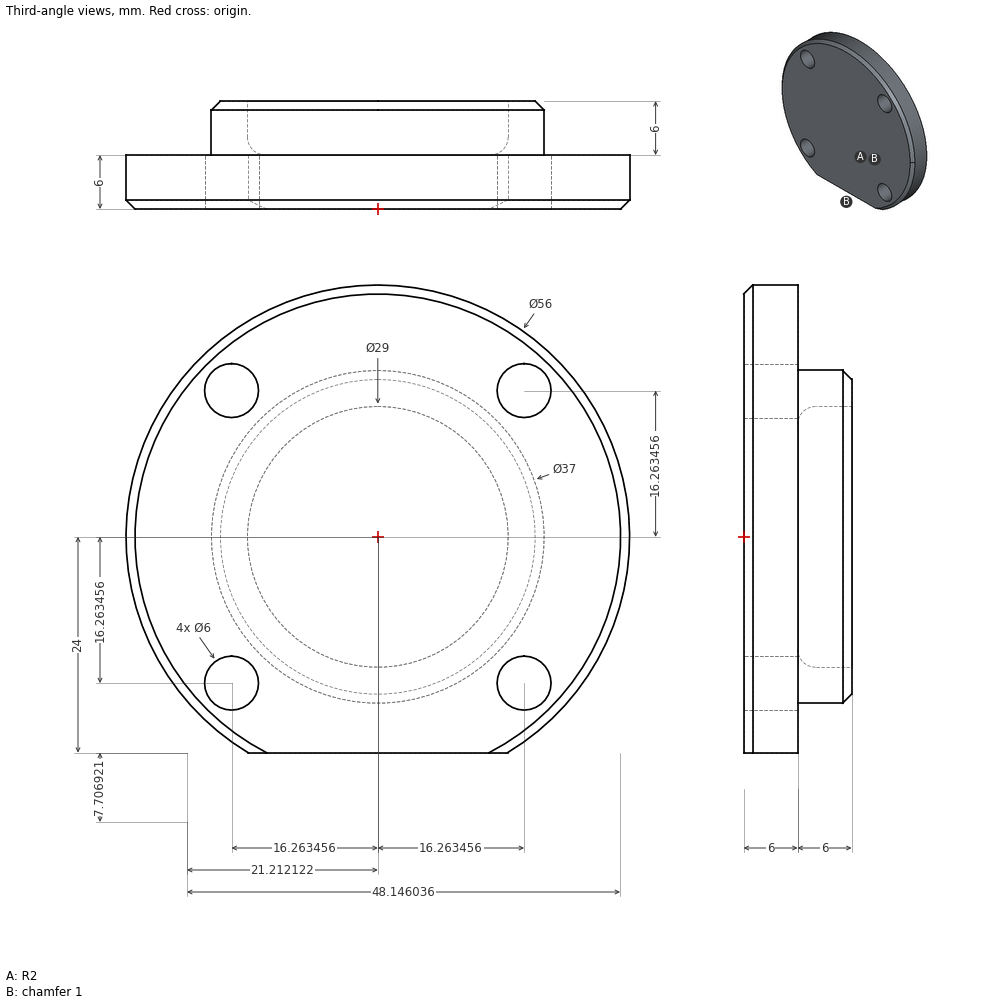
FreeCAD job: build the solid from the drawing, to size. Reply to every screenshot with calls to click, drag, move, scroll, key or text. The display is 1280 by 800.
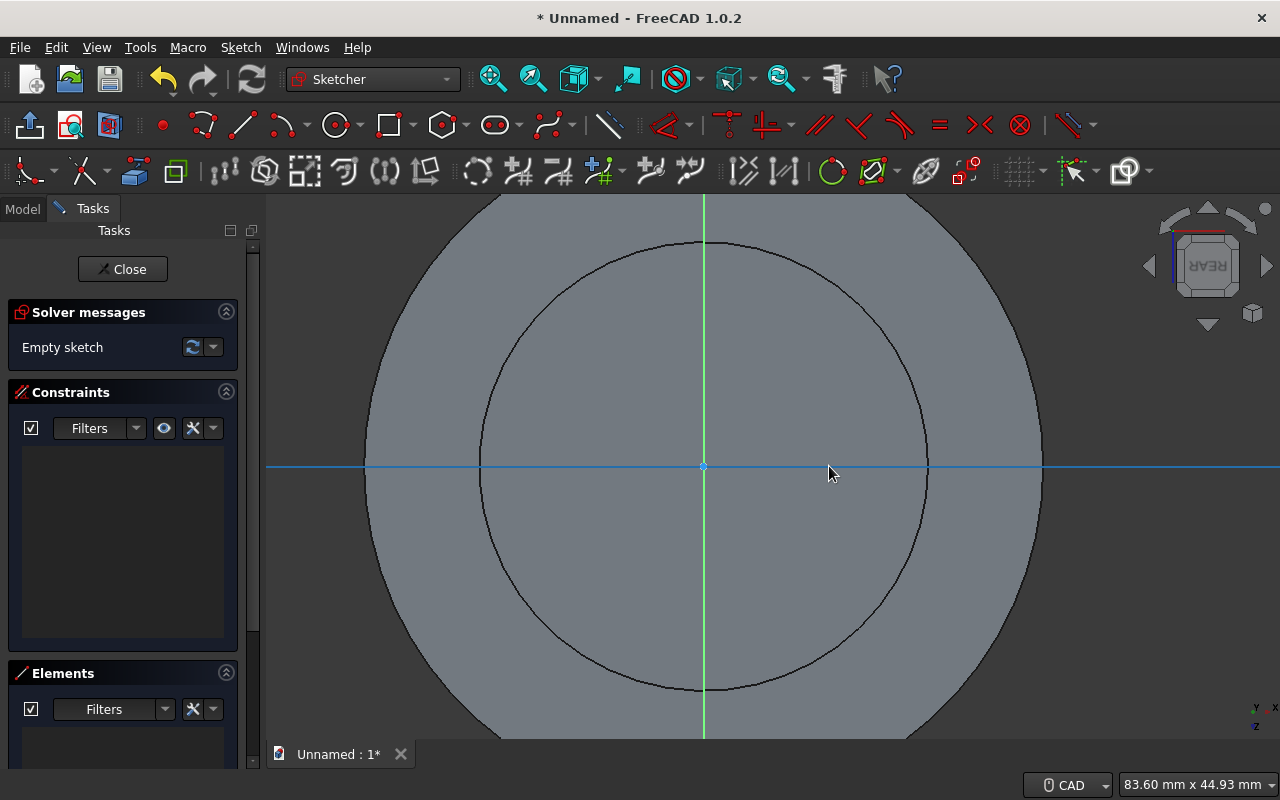
key(g)
key(c)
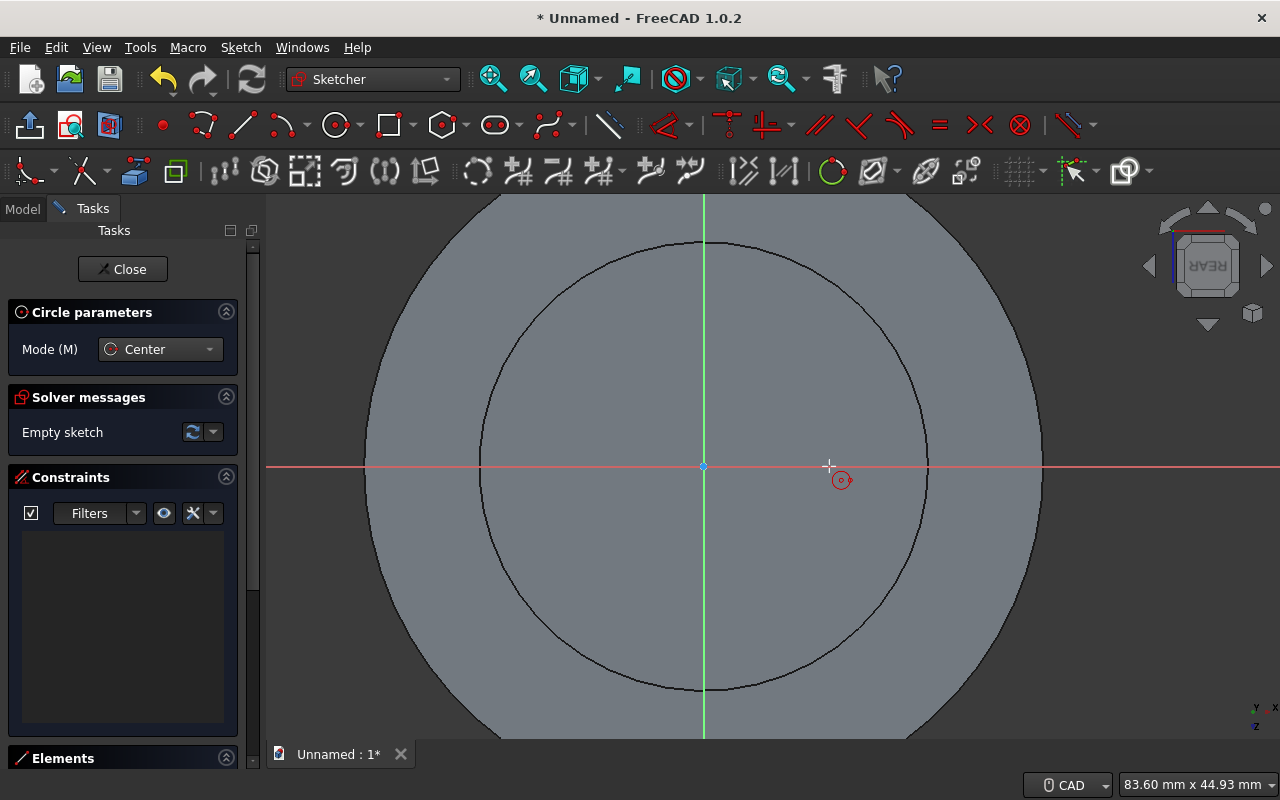
click(704, 466)
click(828, 342)
key(Escape)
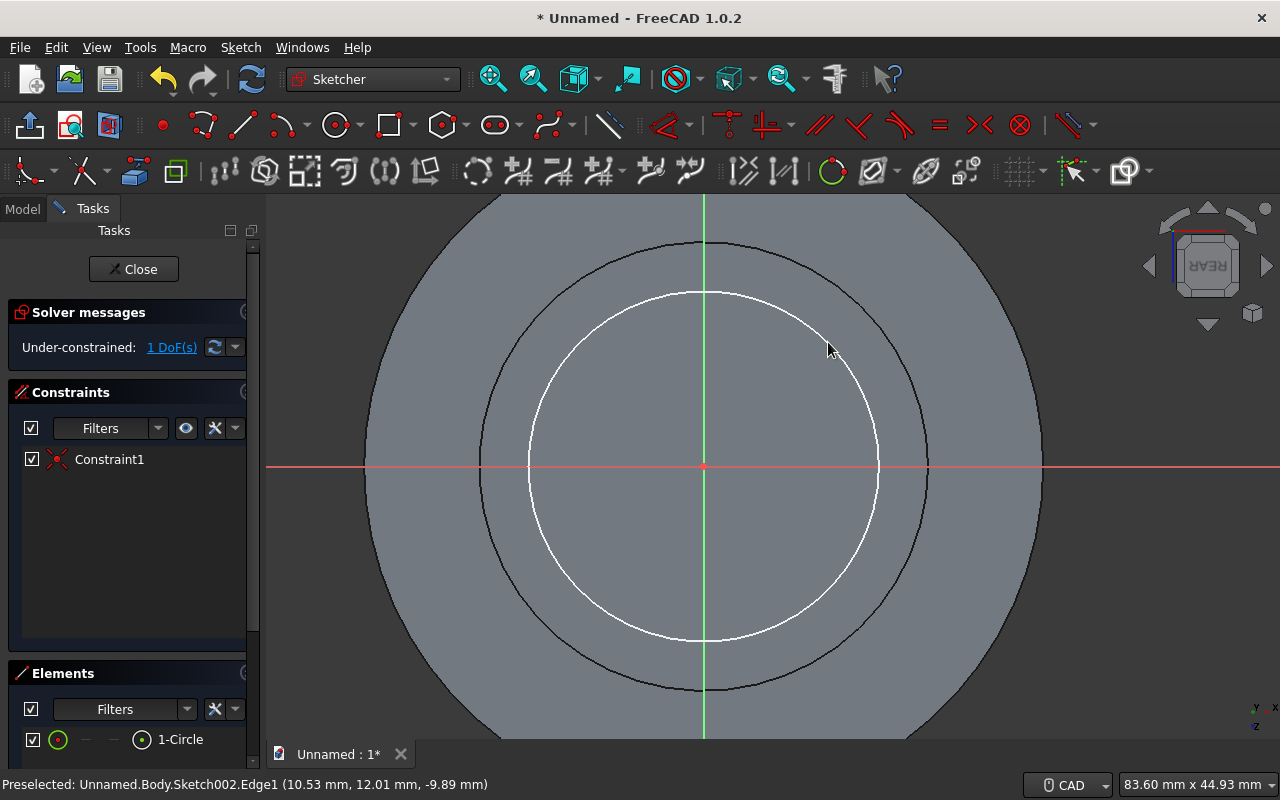
key(d)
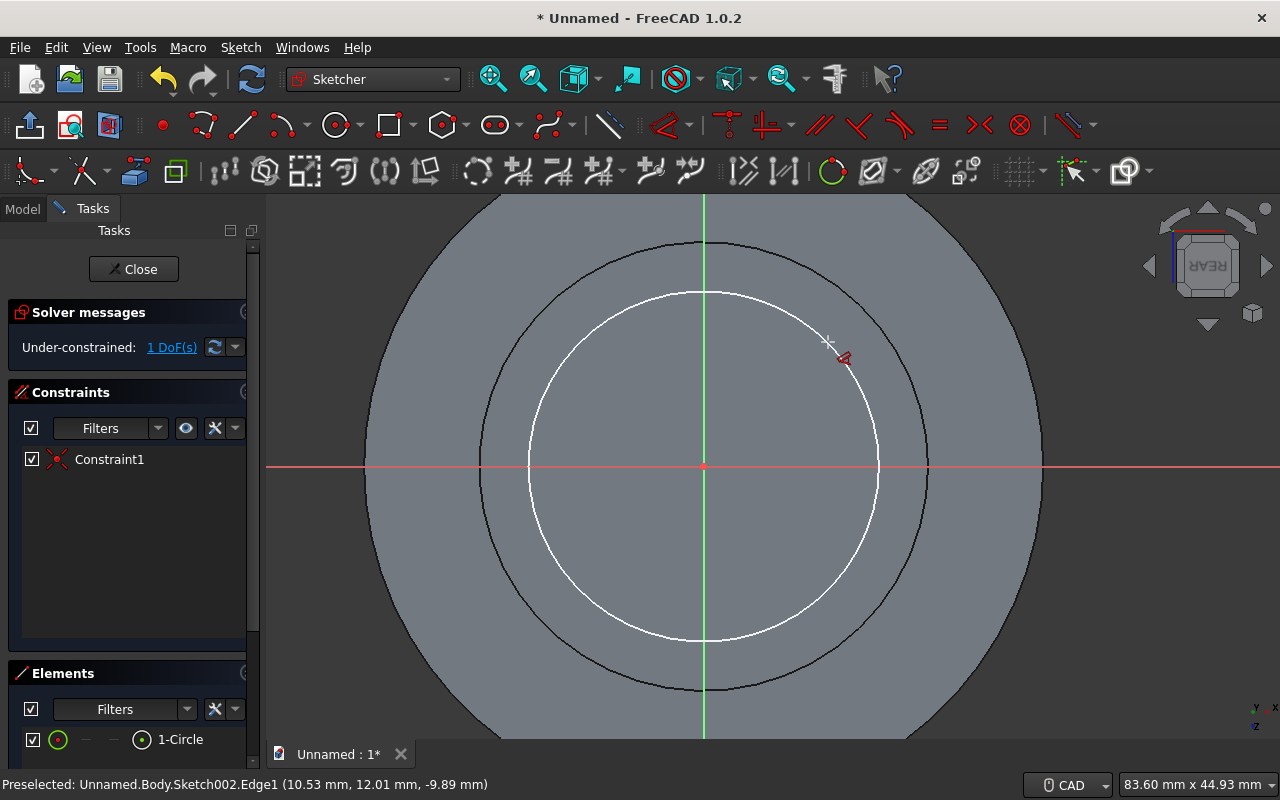
click(827, 342)
click(850, 319)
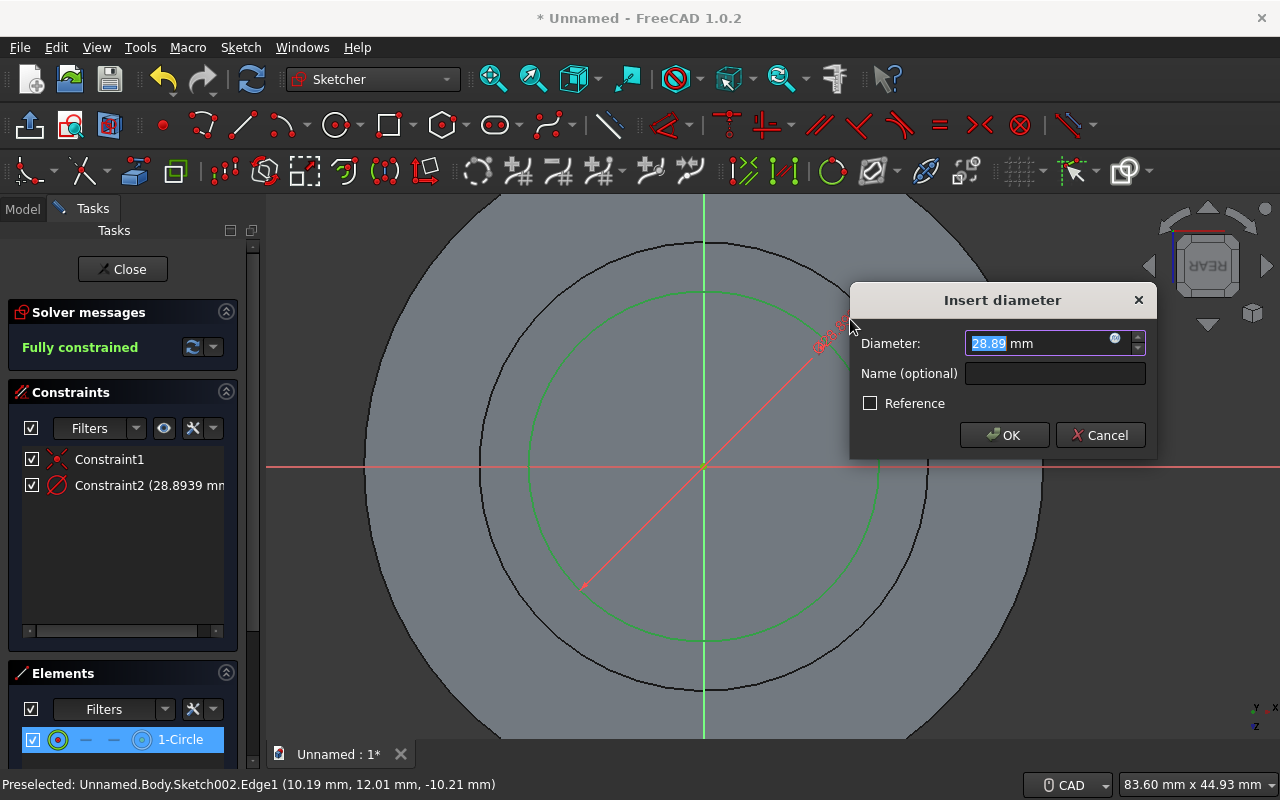
text(29)
key(Return)
key(Escape)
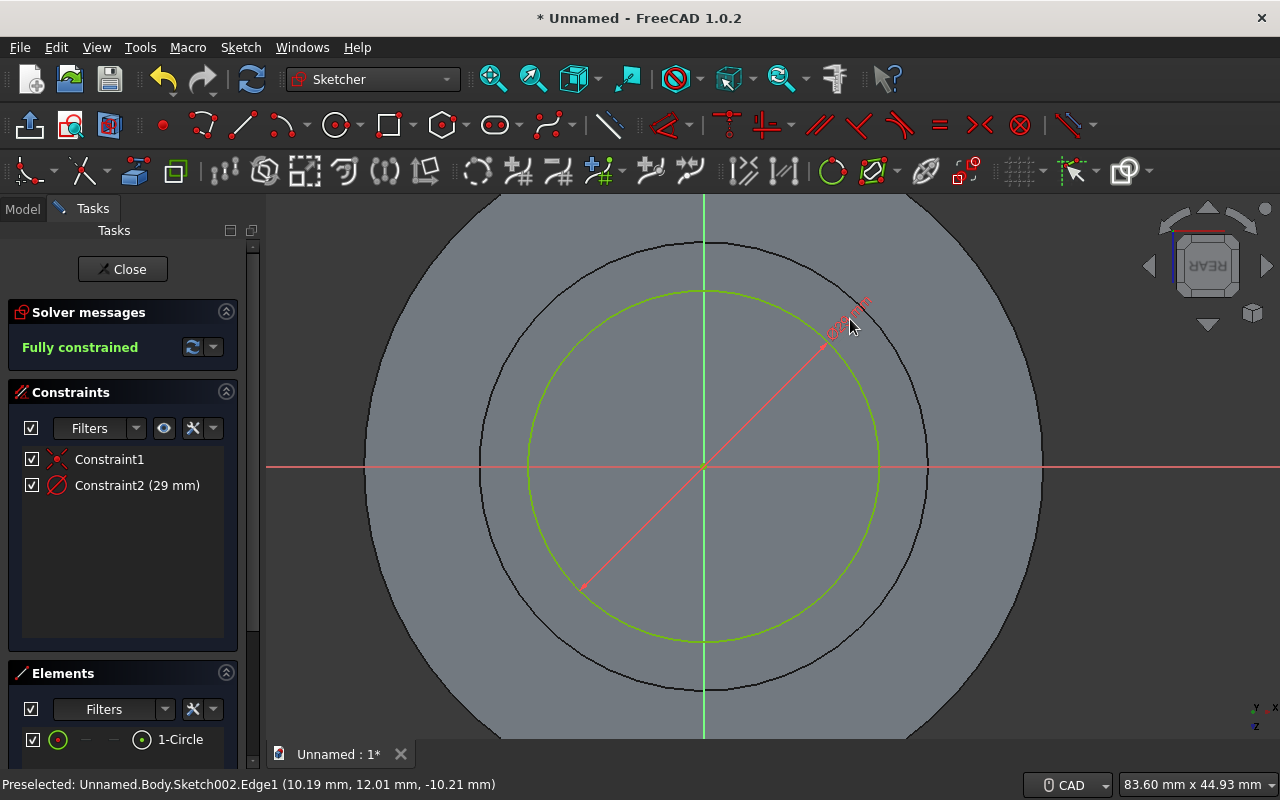
click(123, 269)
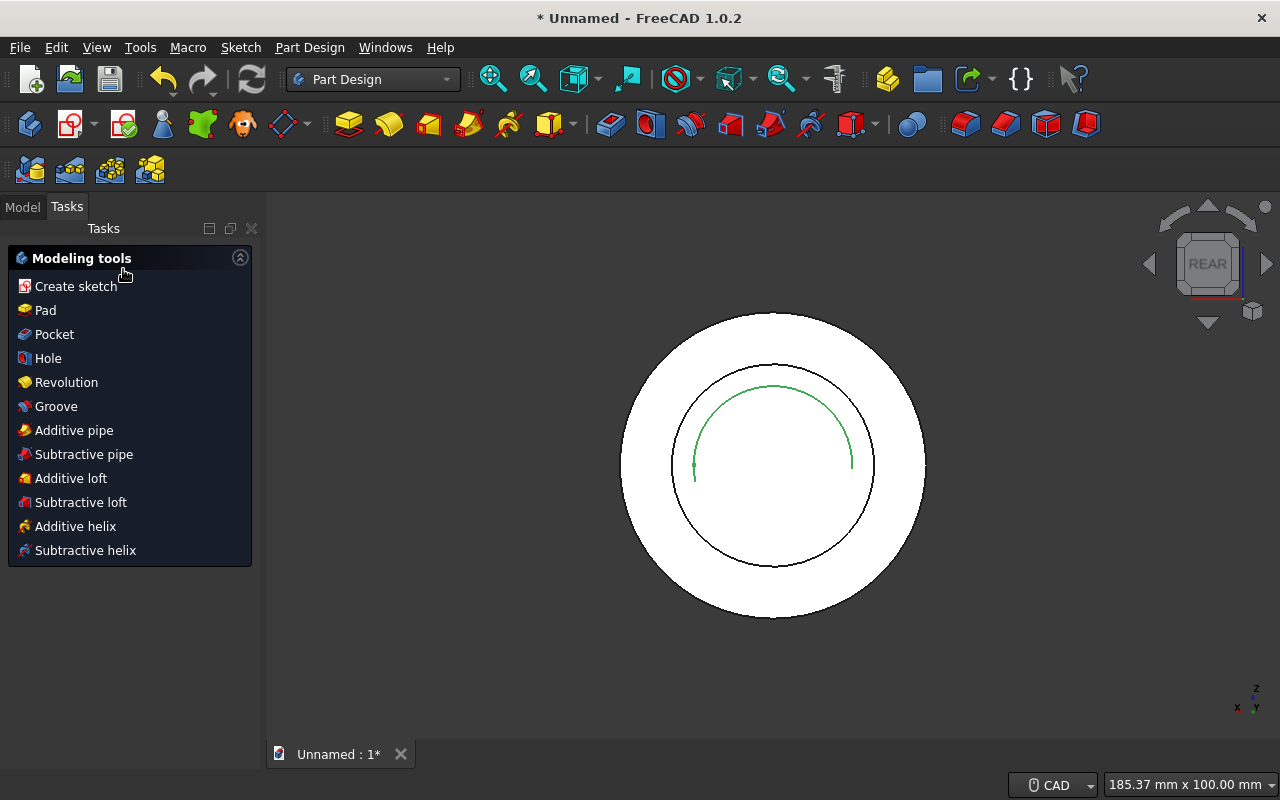
click(612, 124)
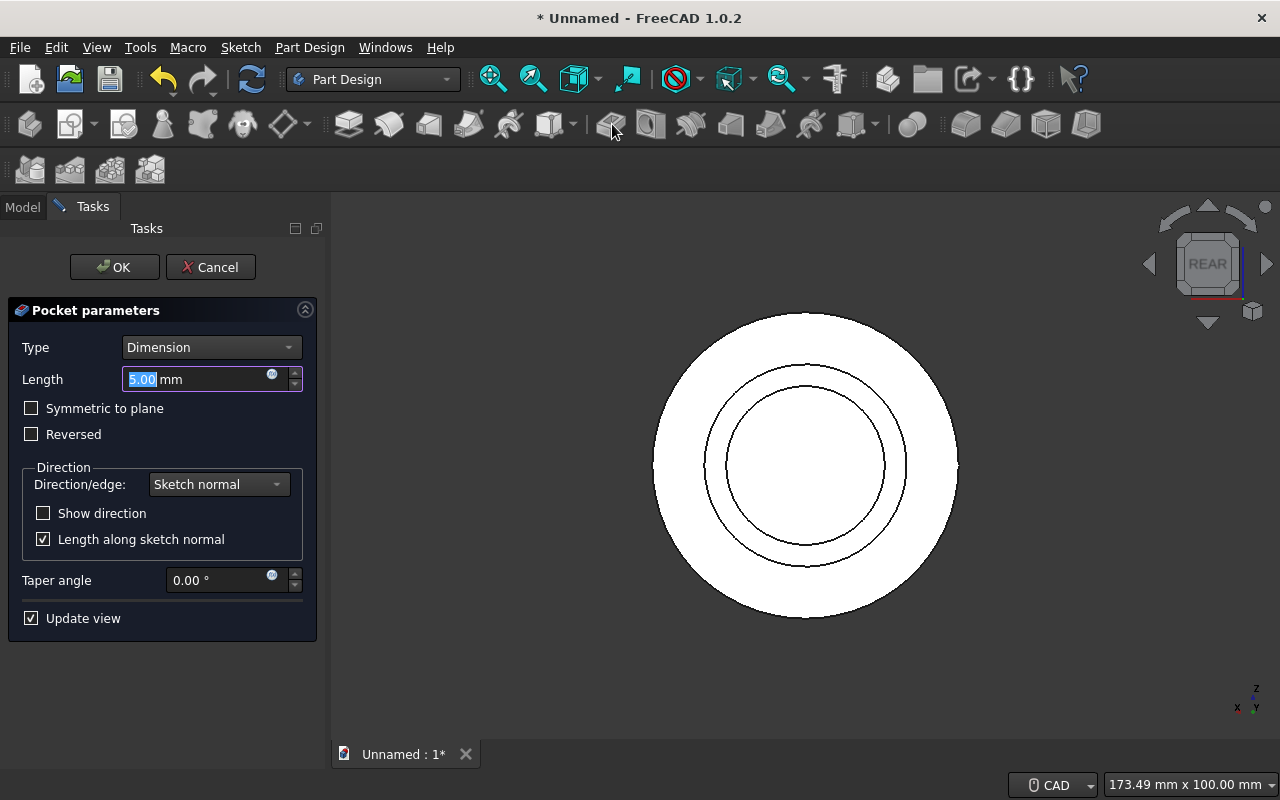
text(6)
key(Tab)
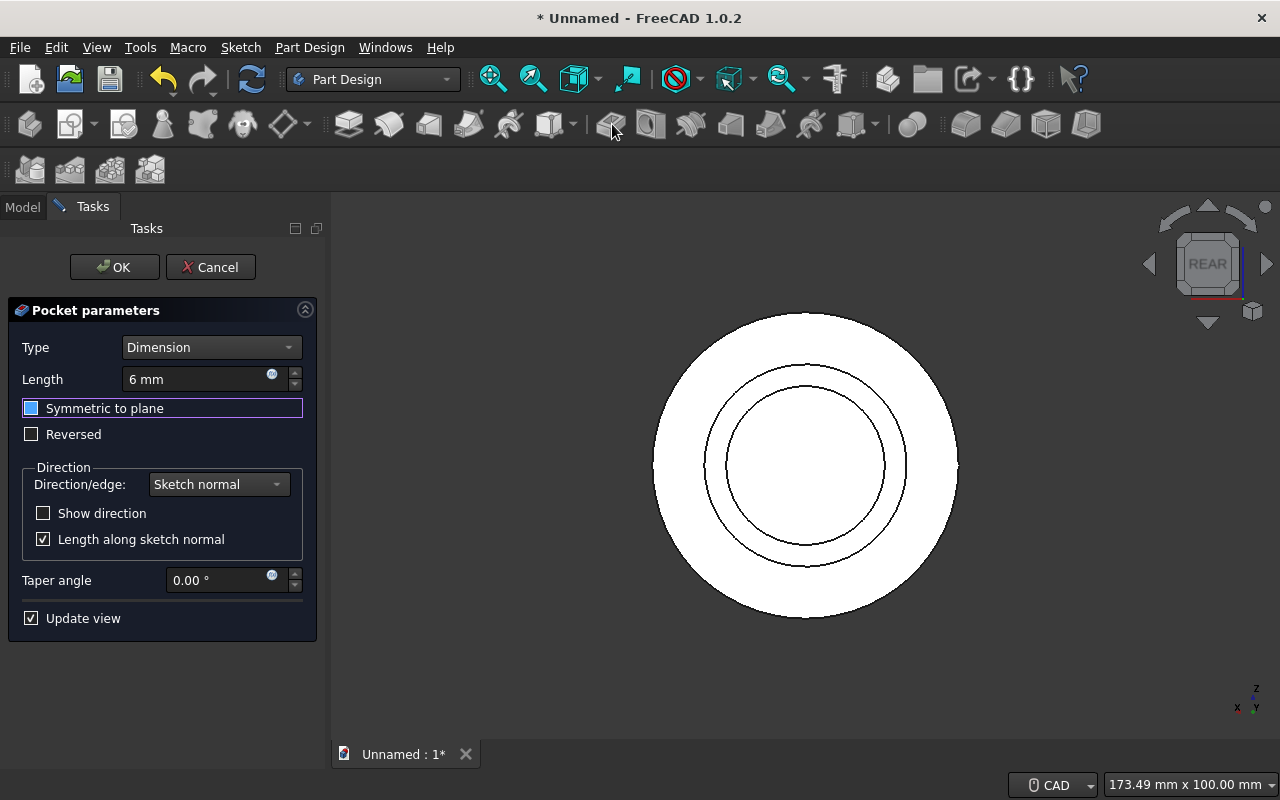
click(115, 267)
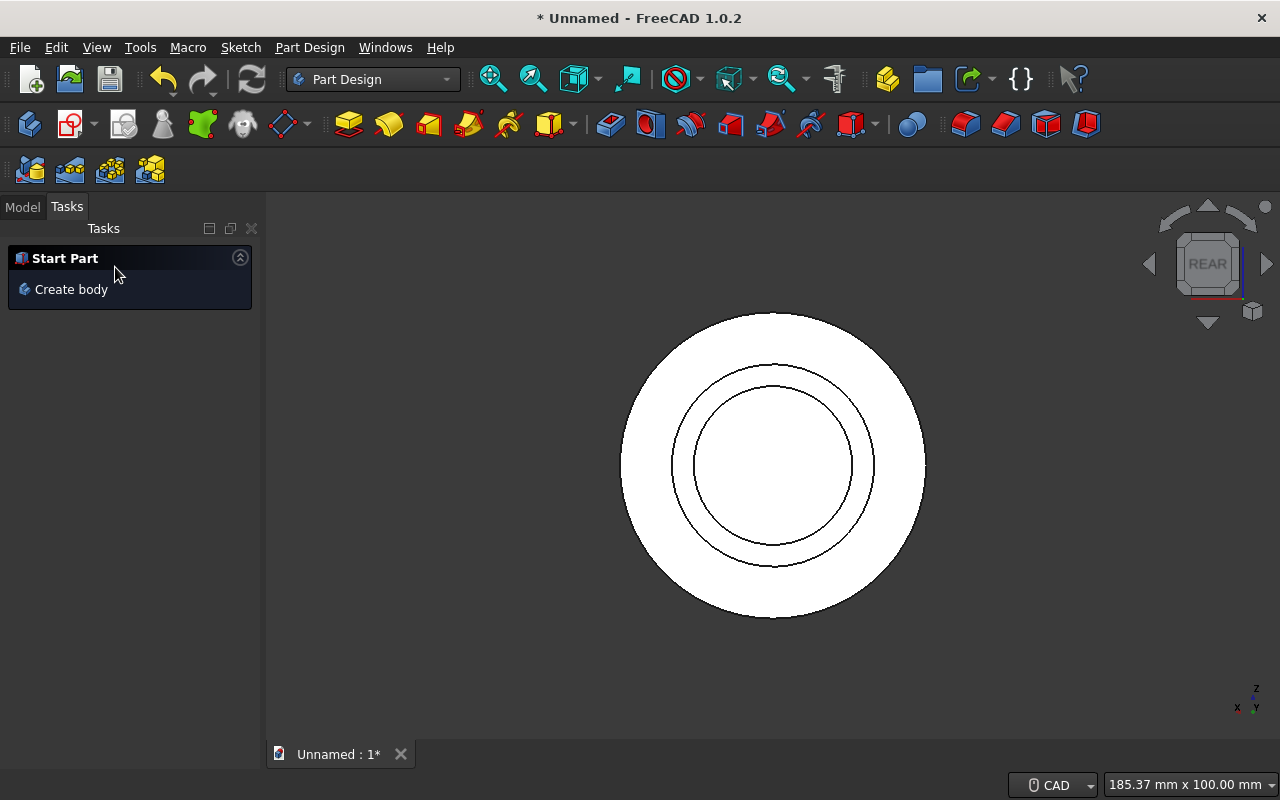
key(0)